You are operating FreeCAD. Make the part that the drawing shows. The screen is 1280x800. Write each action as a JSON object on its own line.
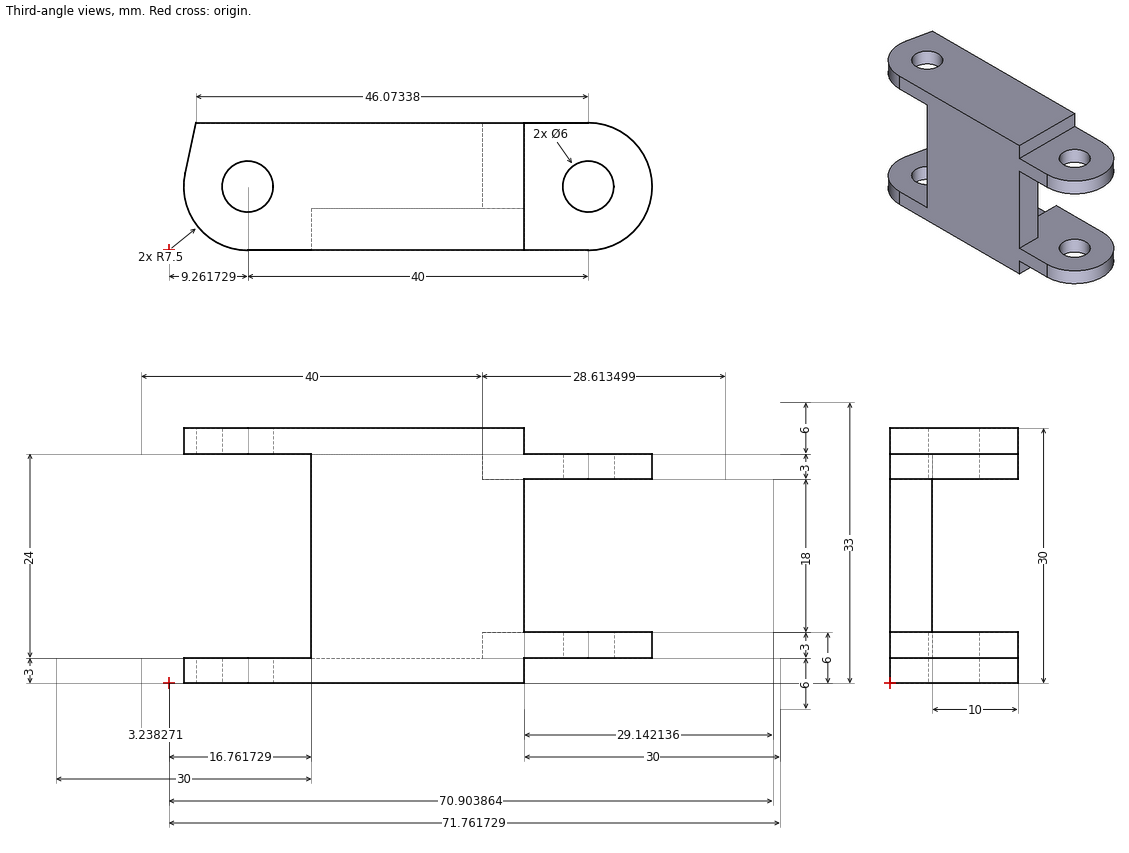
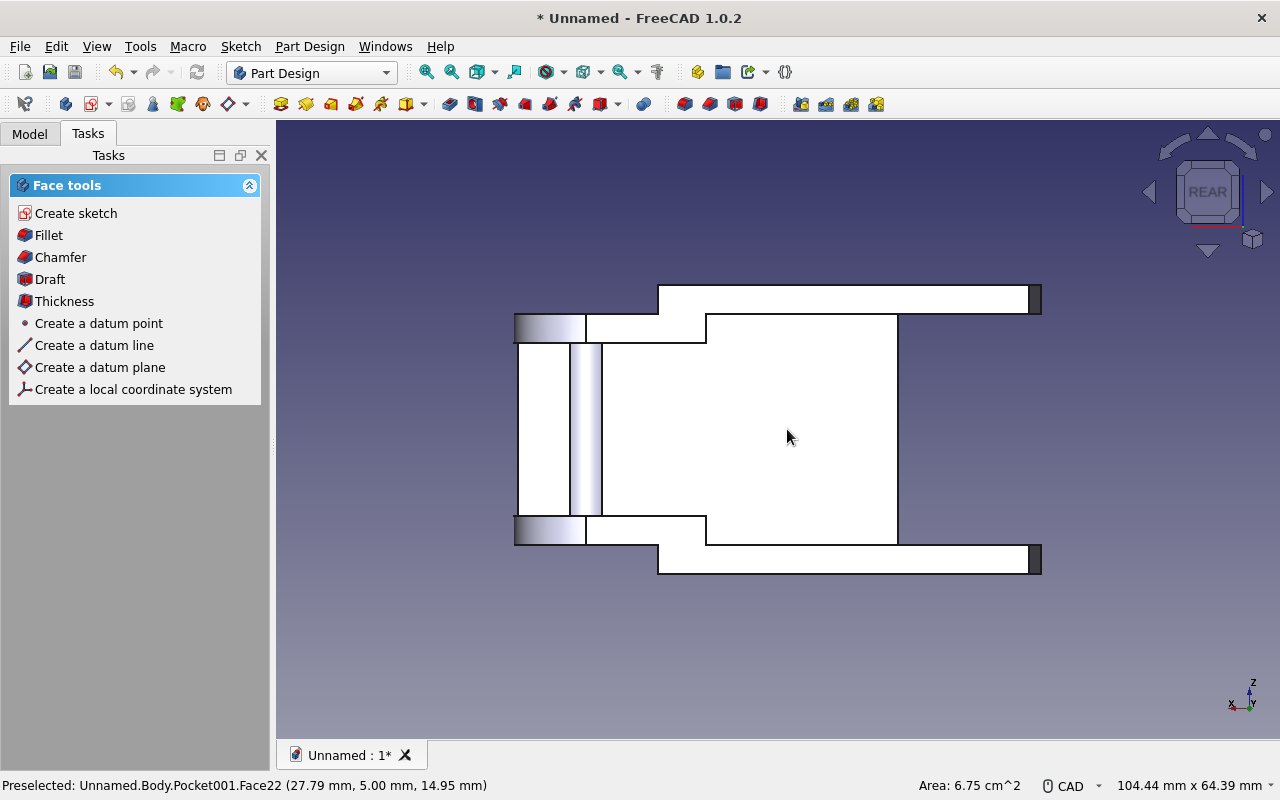
{"action": "left_click", "coordinate": [90, 104]}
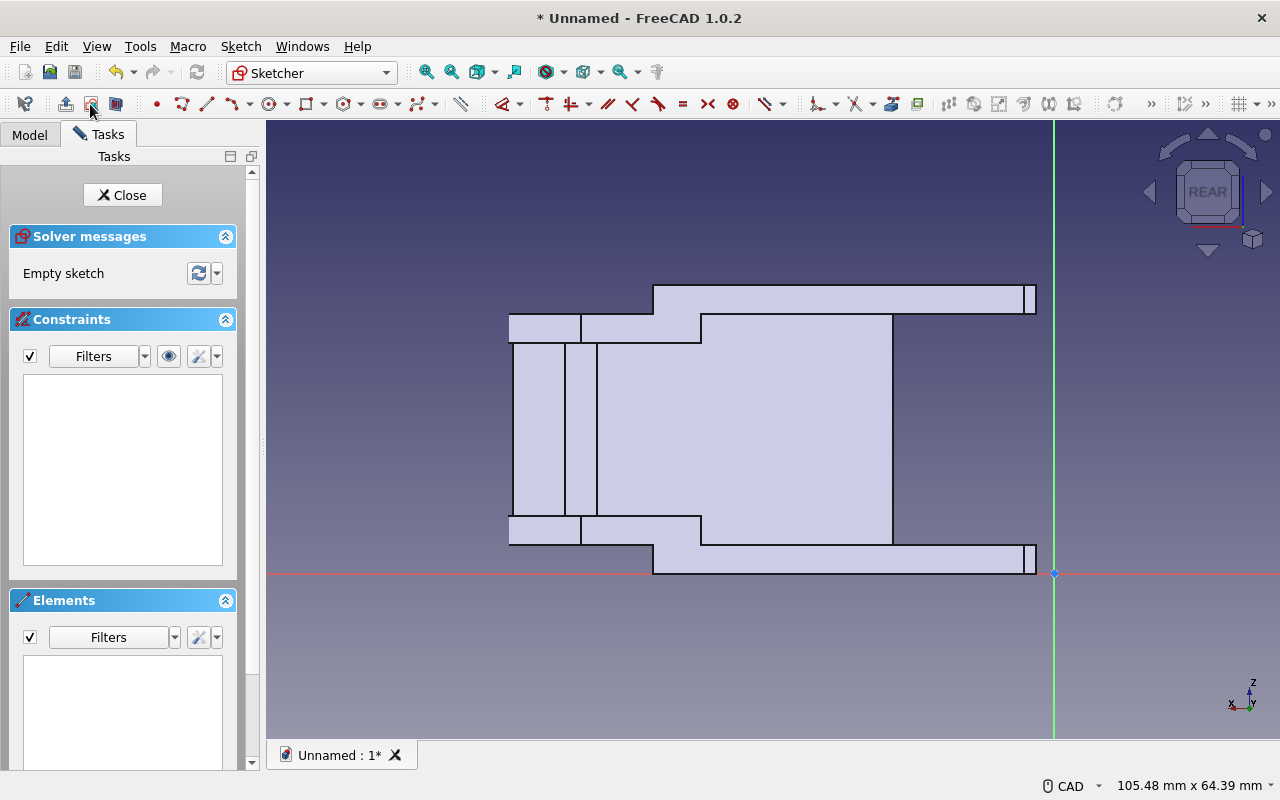
{"action": "left_click", "coordinate": [306, 104]}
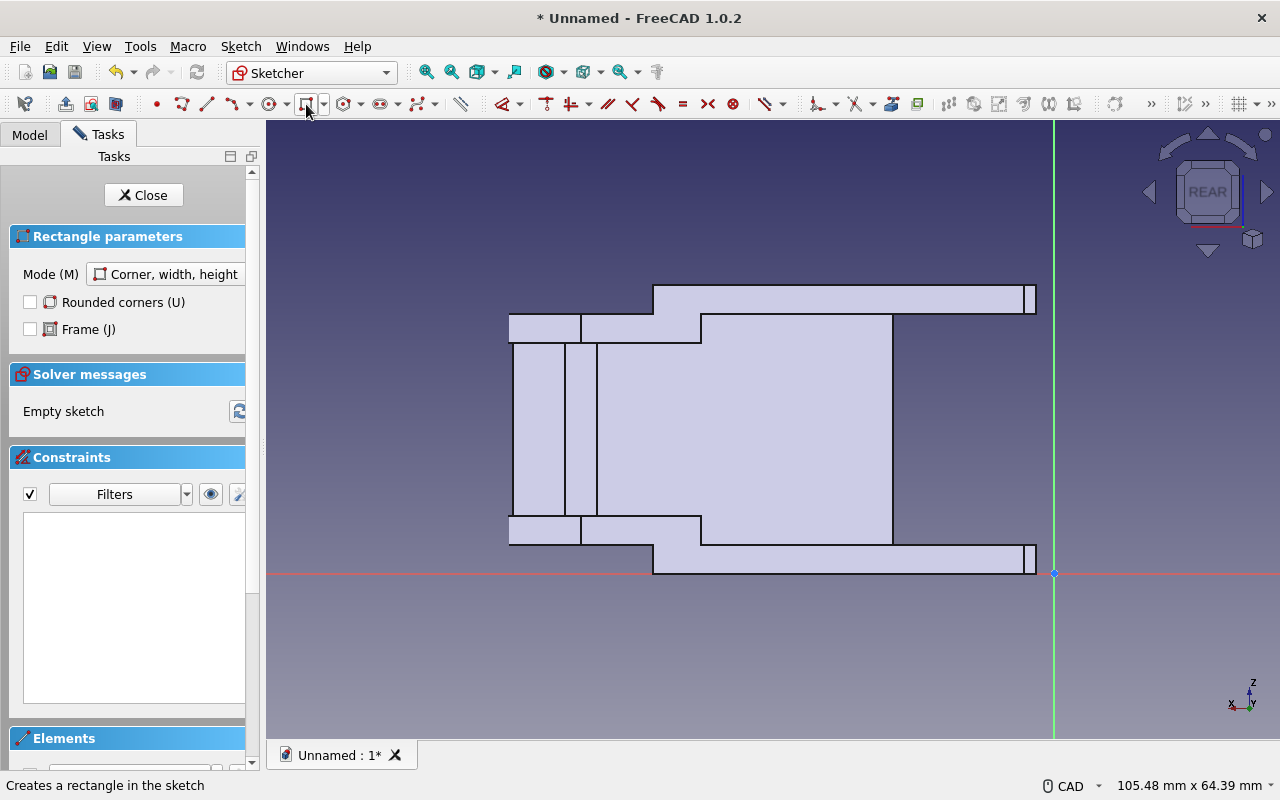
{"action": "left_click", "coordinate": [373, 343]}
{"action": "left_click", "coordinate": [653, 516]}
{"action": "key", "text": "Escape"}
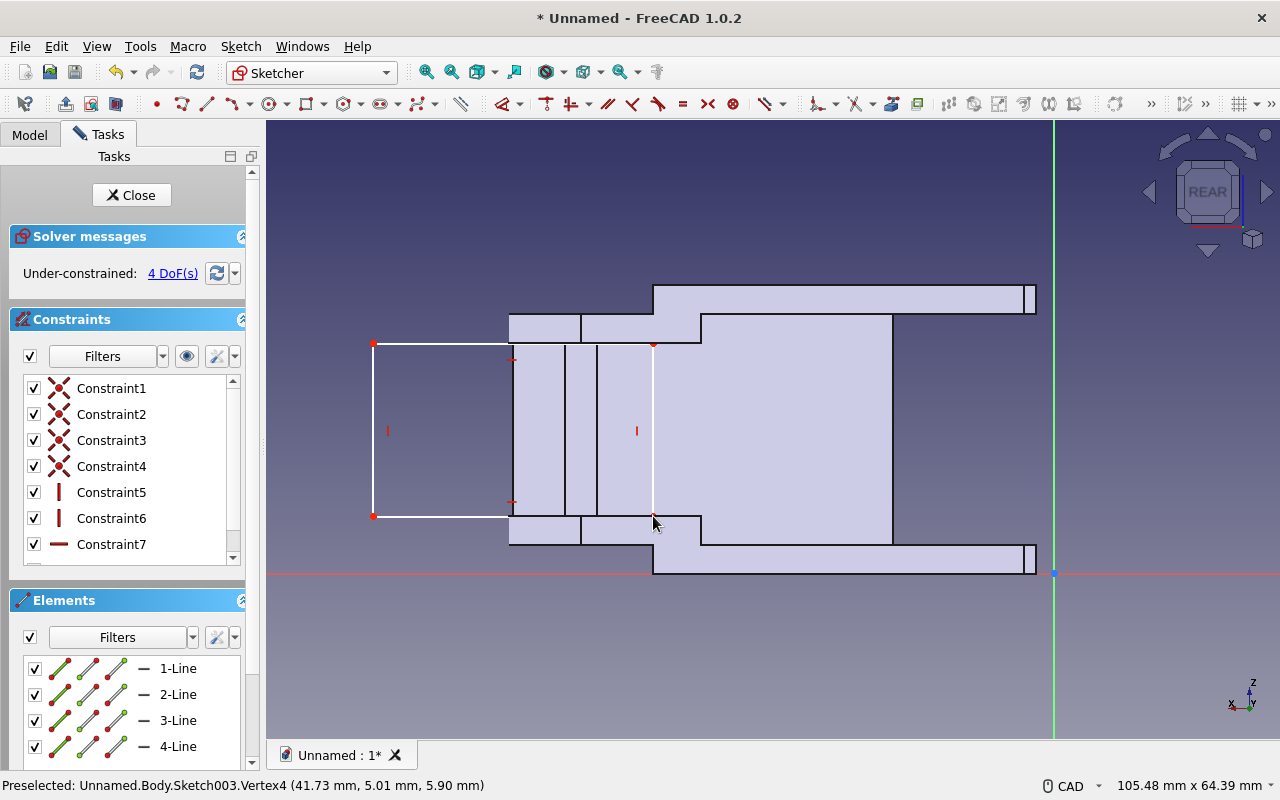
{"action": "left_click", "coordinate": [502, 104]}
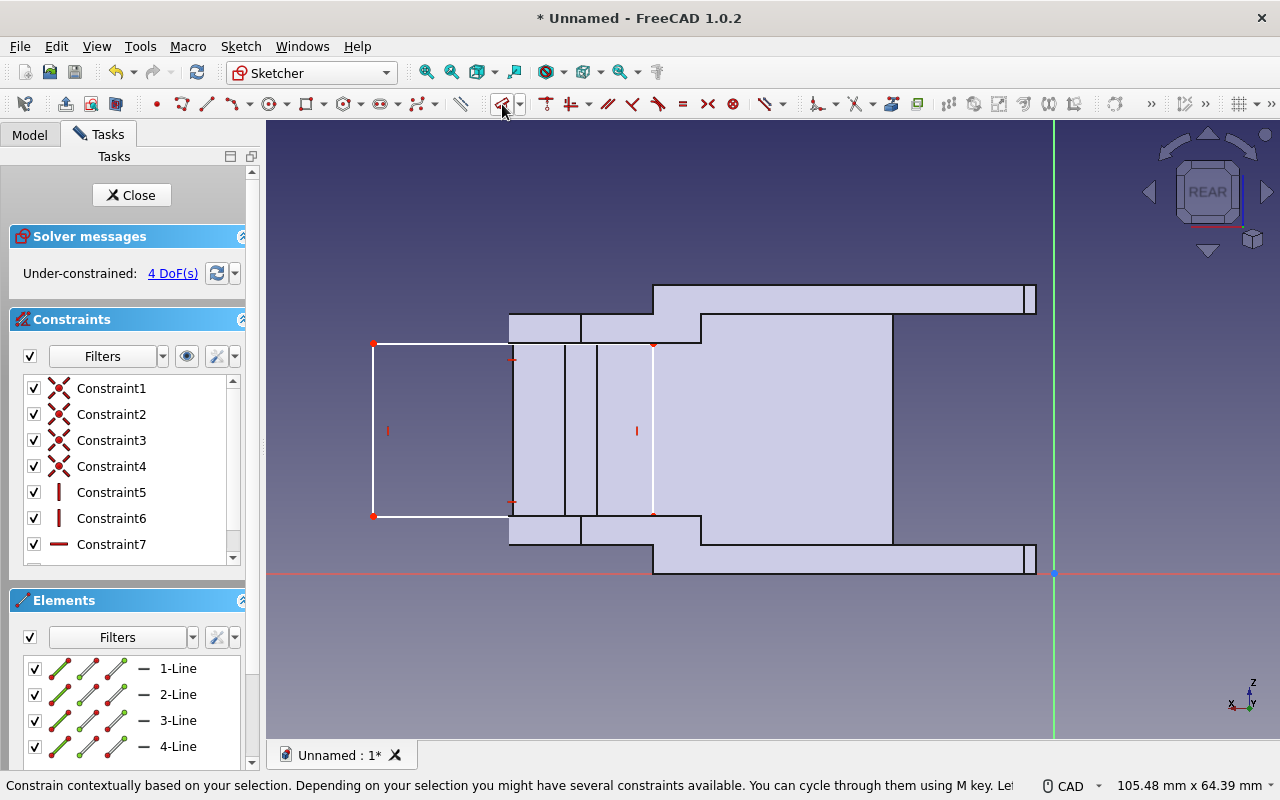
{"action": "left_click", "coordinate": [373, 396]}
{"action": "left_click", "coordinate": [339, 430]}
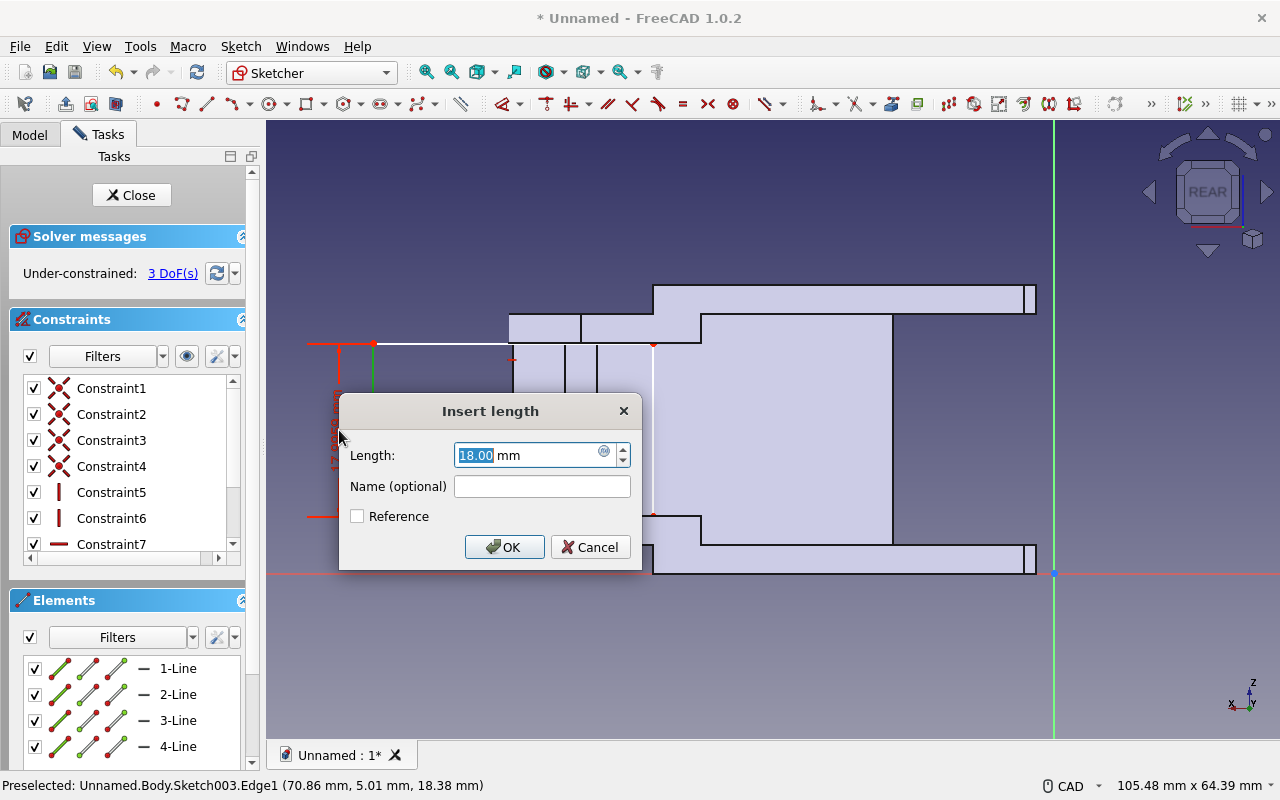
{"action": "type", "text": "18"}
{"action": "key", "text": "Return"}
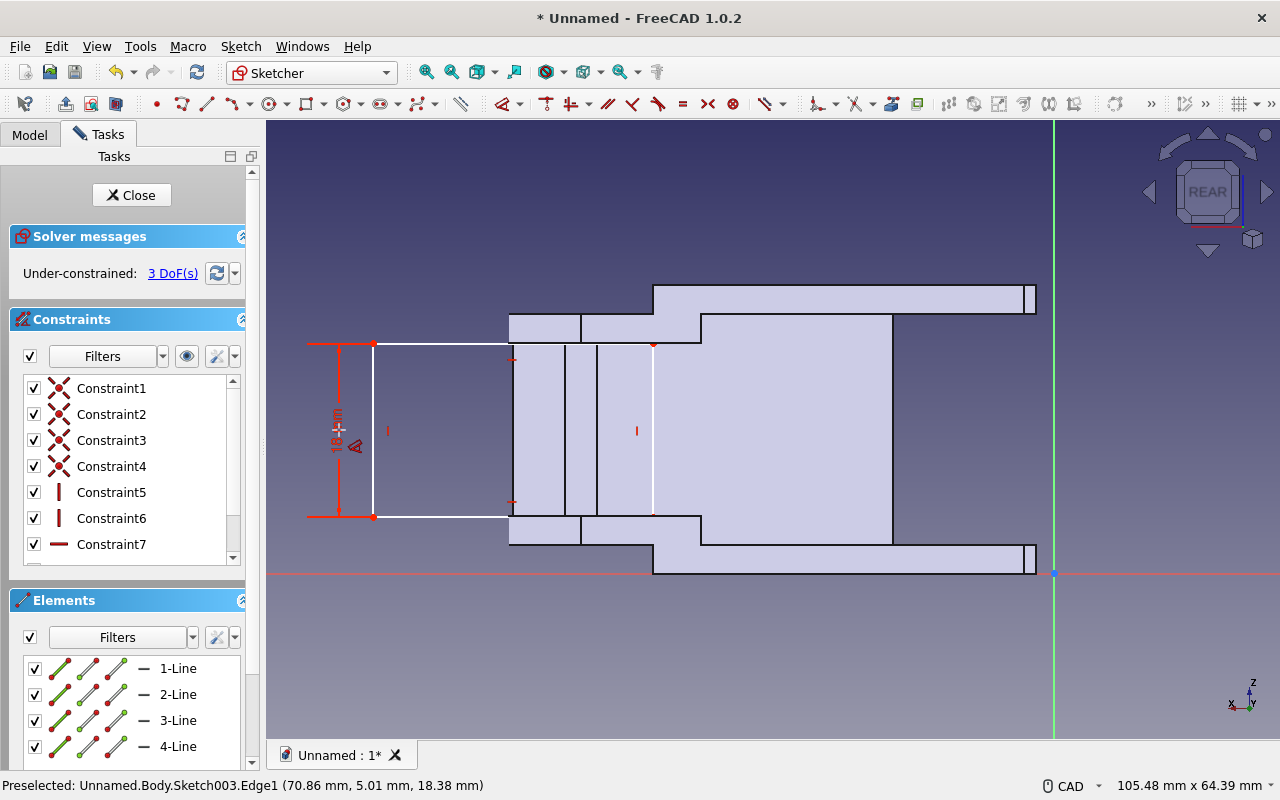
{"action": "left_click", "coordinate": [373, 517]}
{"action": "left_click", "coordinate": [1088, 545]}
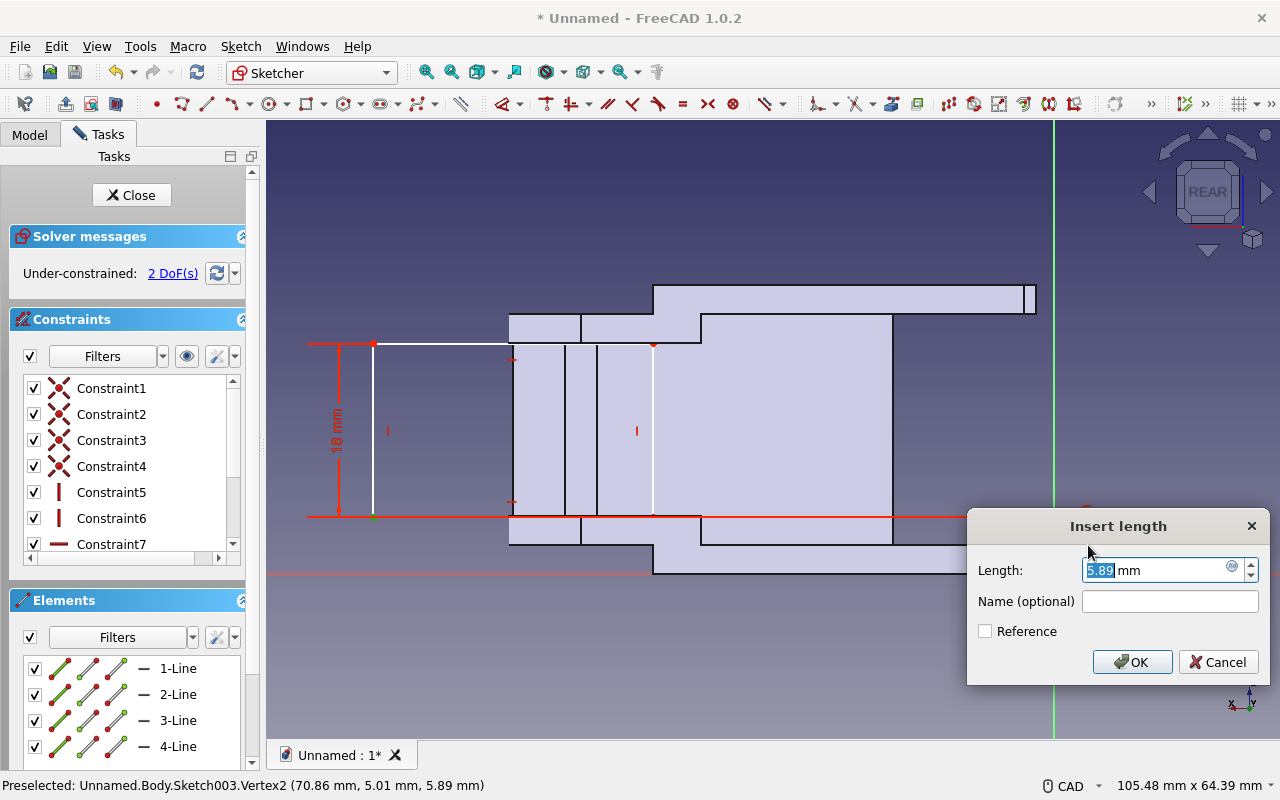
{"action": "type", "text": "6"}
{"action": "key", "text": "Return"}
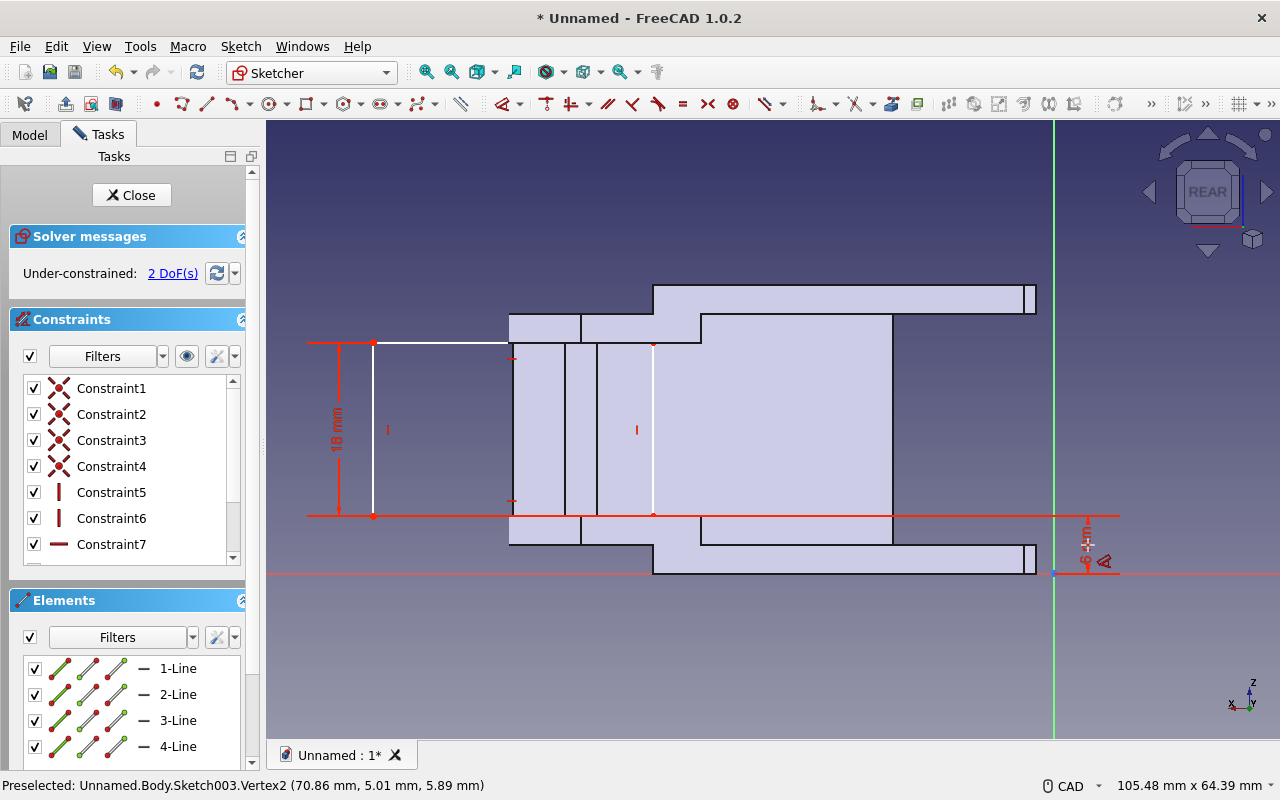
{"action": "left_click", "coordinate": [457, 516]}
{"action": "left_click", "coordinate": [513, 550]}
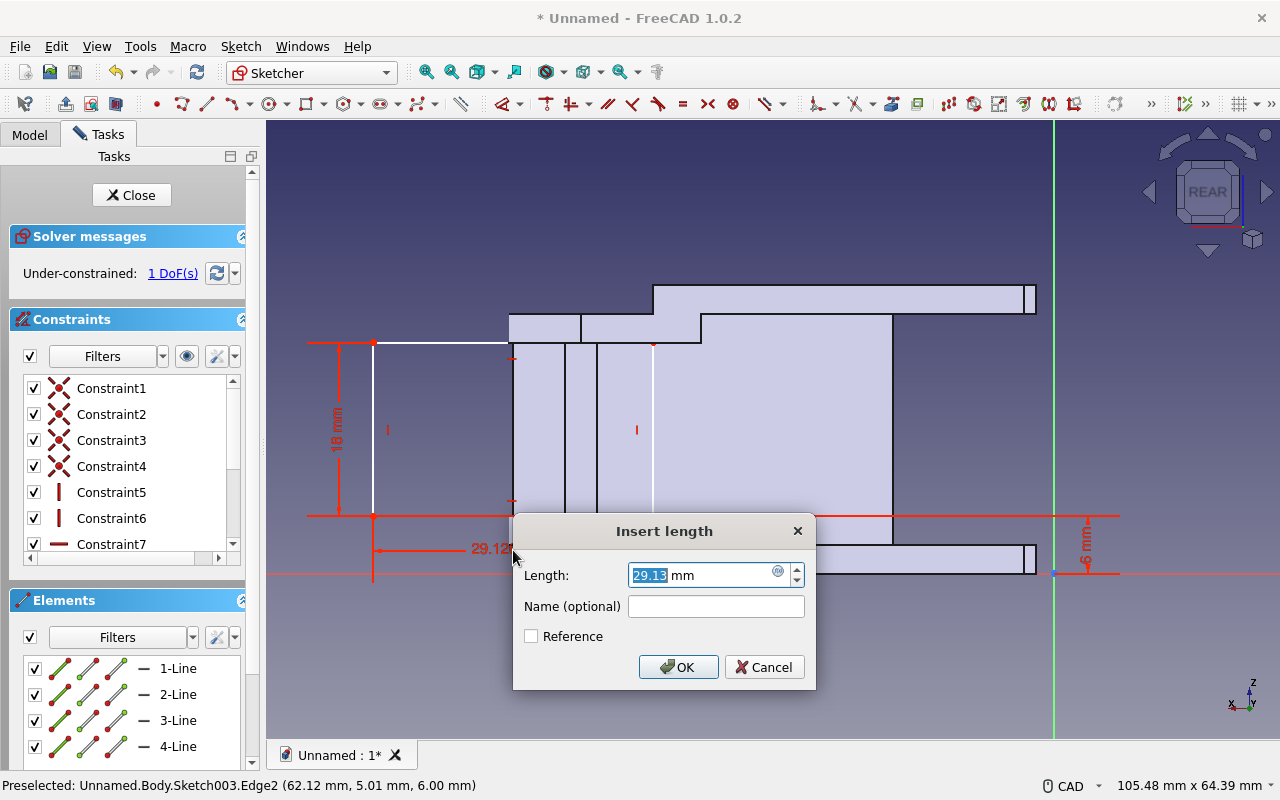
{"action": "type", "text": "29.142136"}
{"action": "key", "text": "Return"}